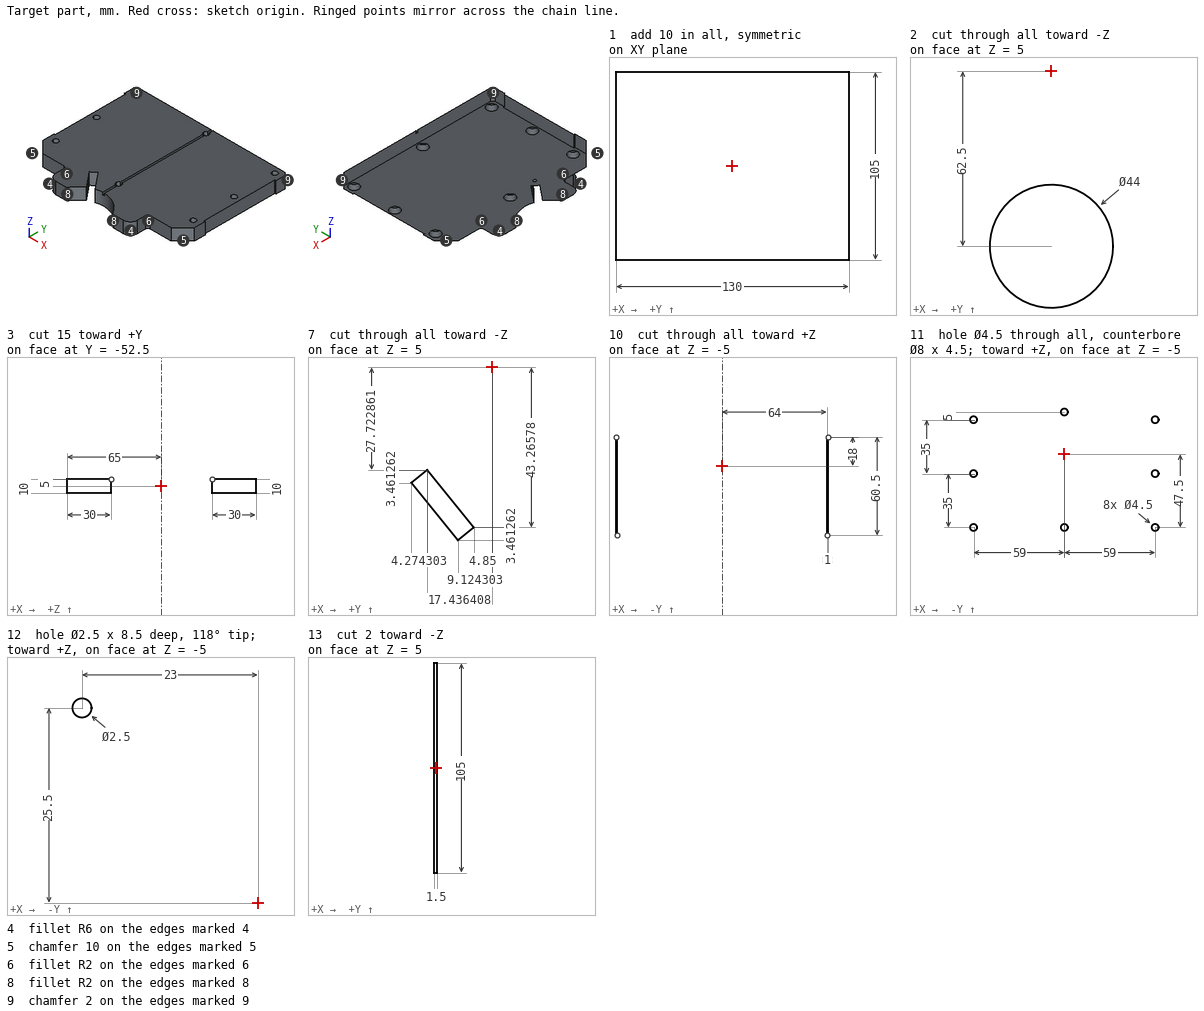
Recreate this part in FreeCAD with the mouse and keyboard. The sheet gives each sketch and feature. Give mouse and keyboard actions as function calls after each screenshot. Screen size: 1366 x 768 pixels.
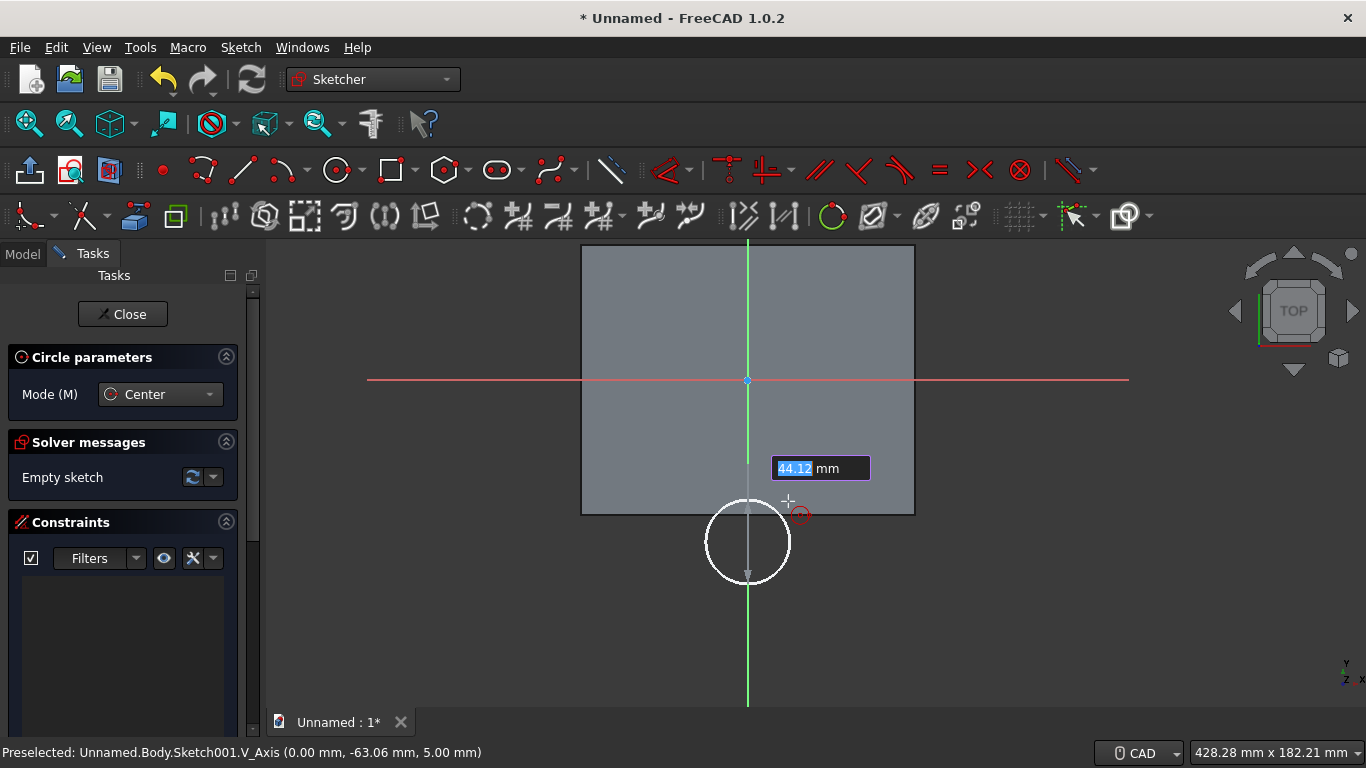
text(44)
key(Return)
key(Escape)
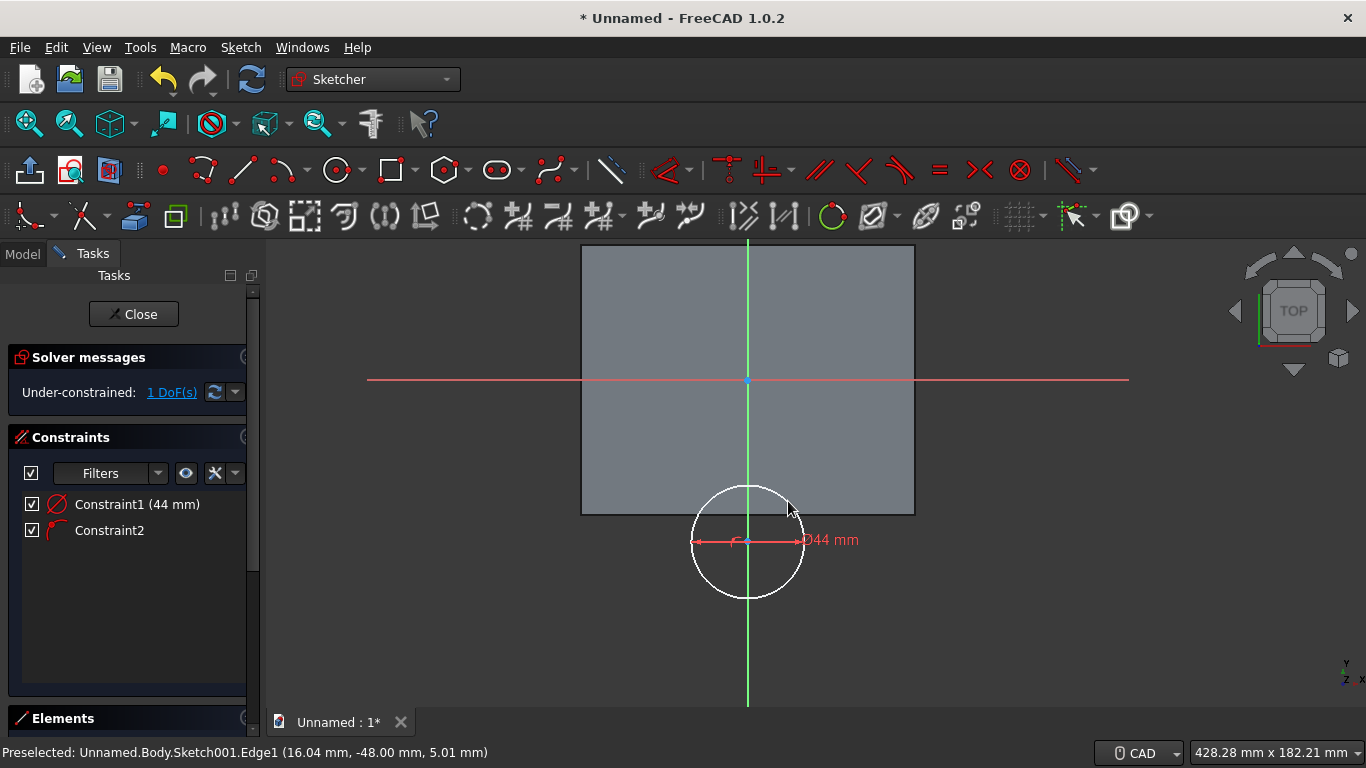
click(666, 170)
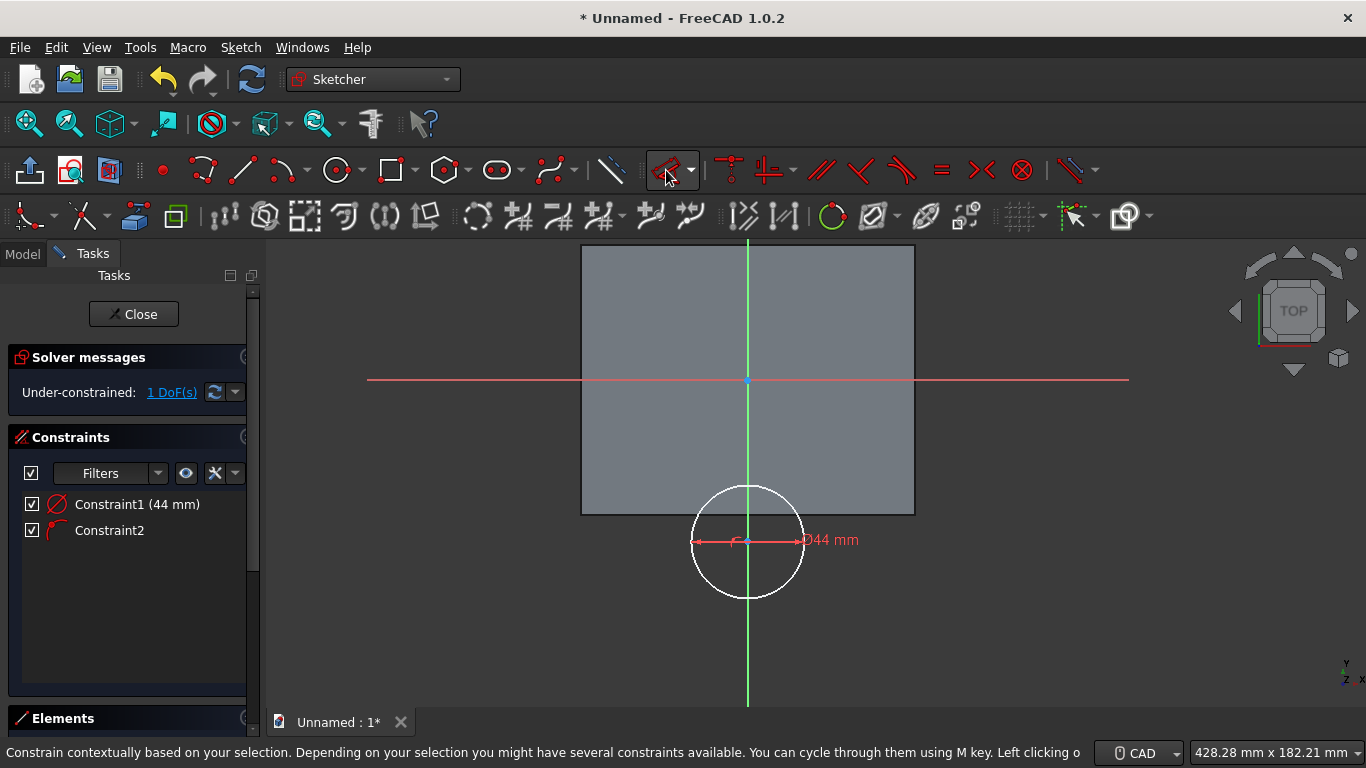
click(748, 542)
click(782, 461)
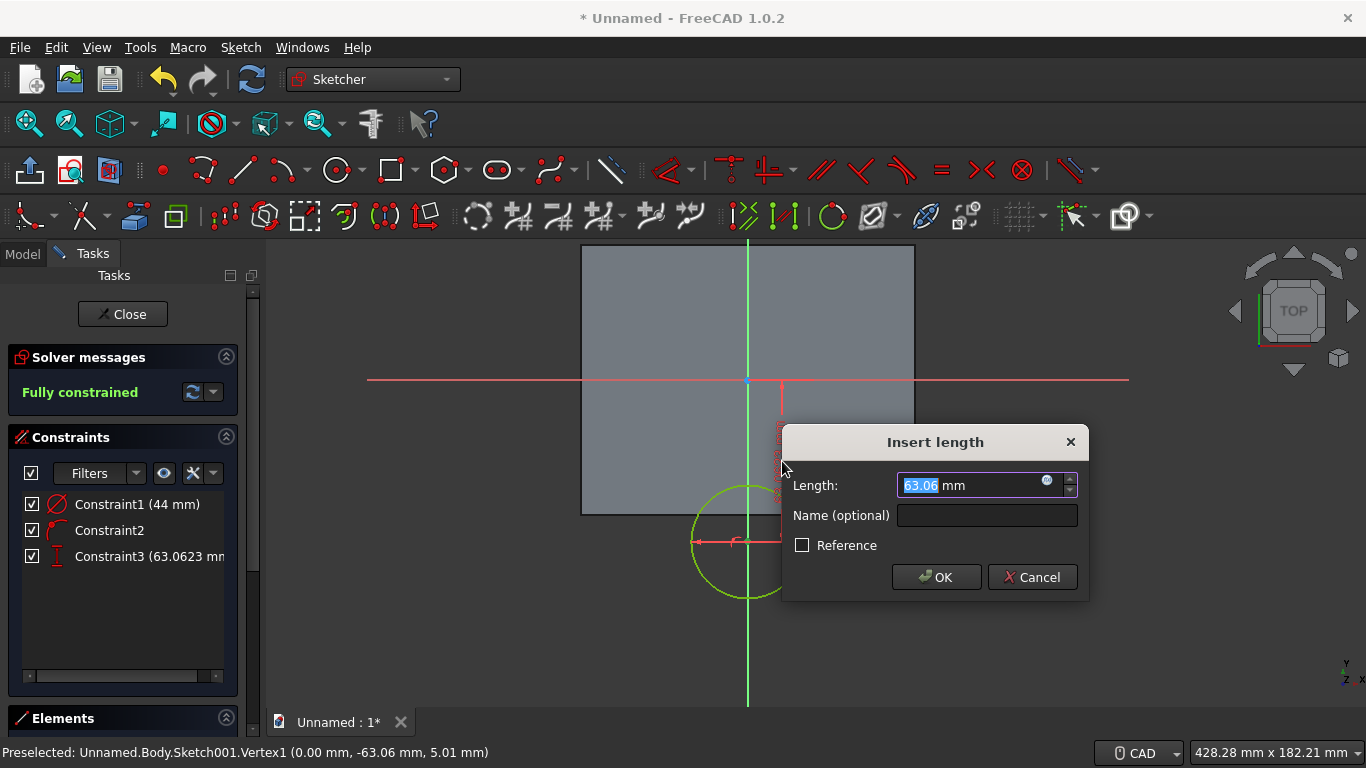
text(62.5)
key(Return)
key(Escape)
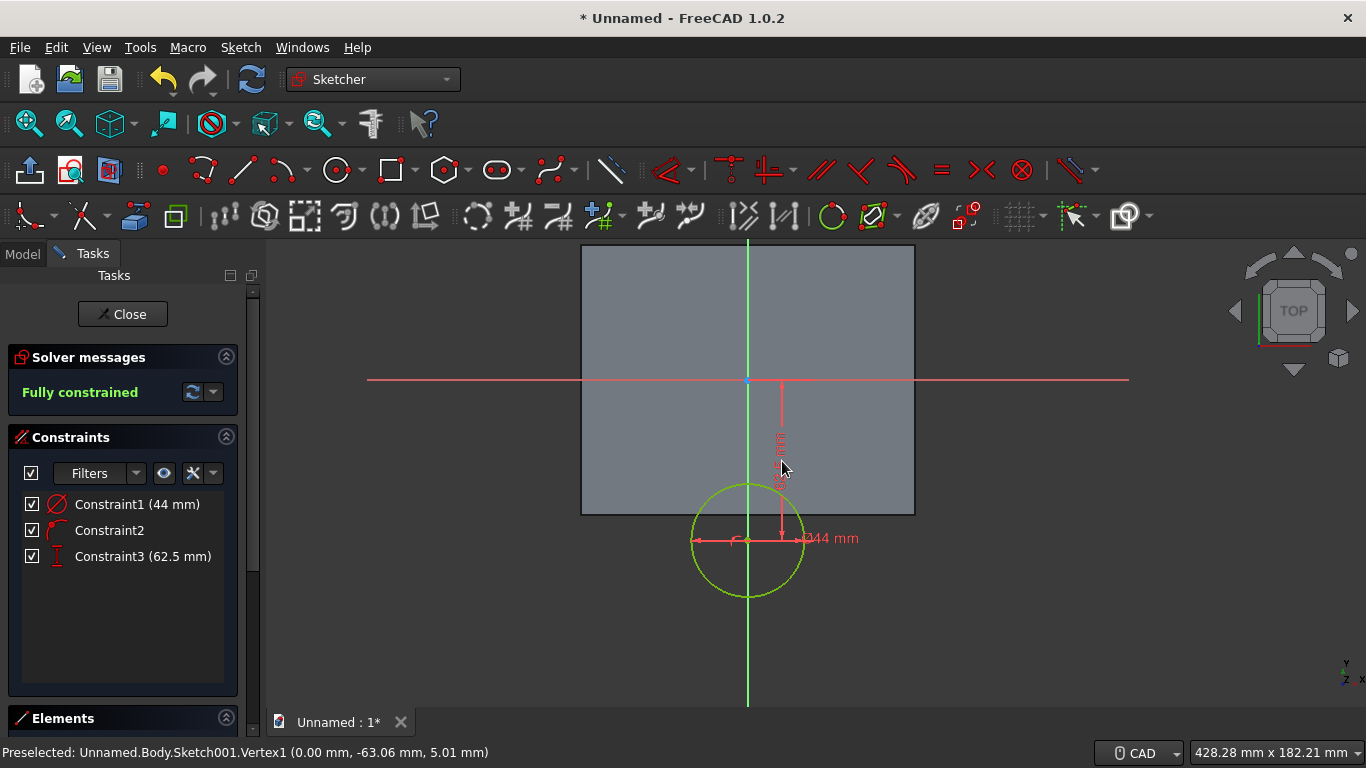
click(123, 314)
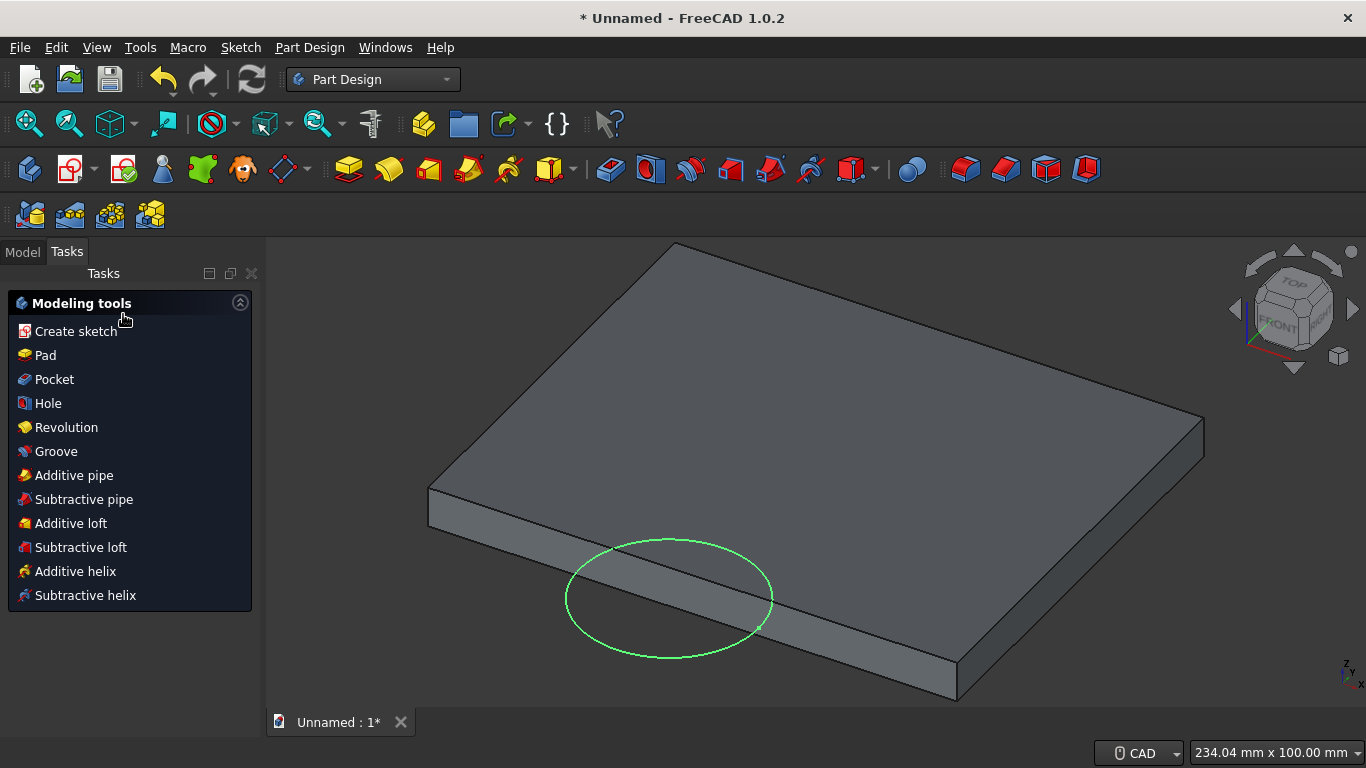
click(612, 170)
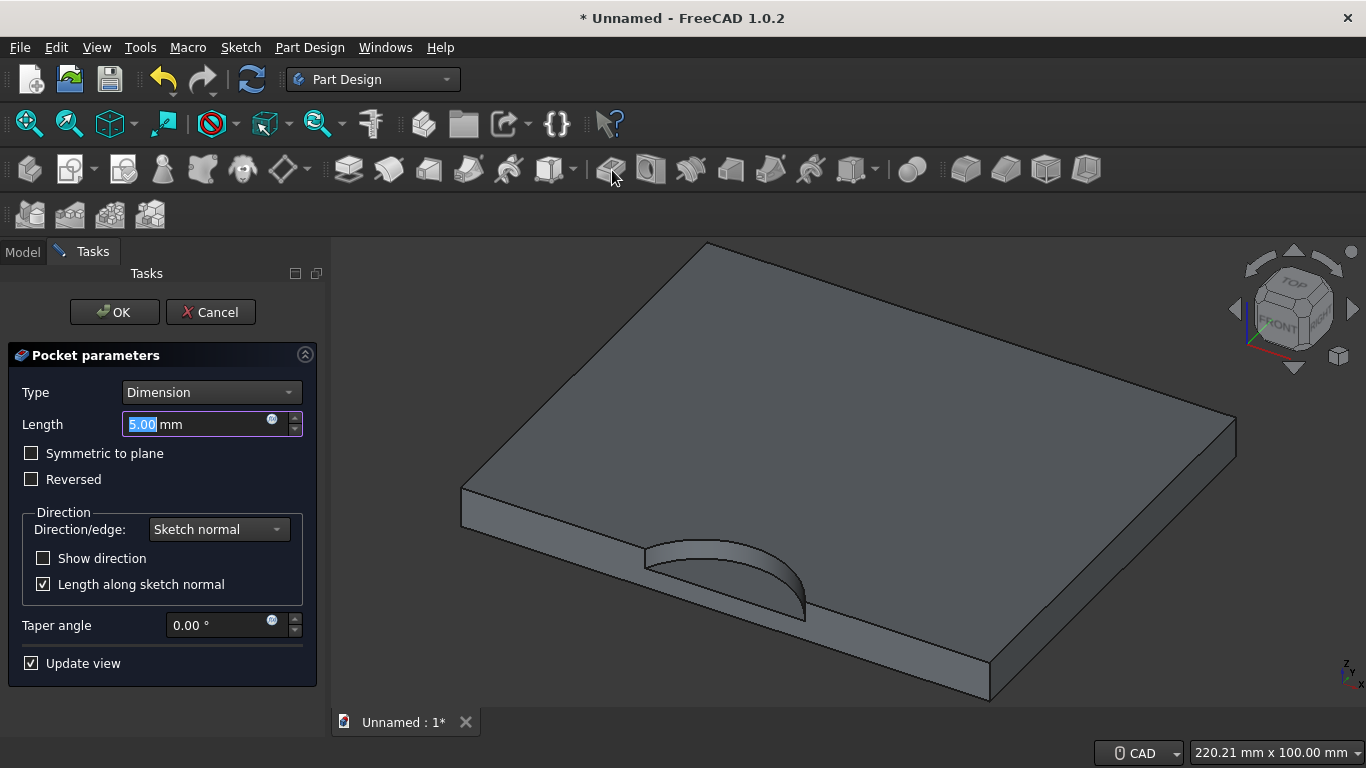
click(212, 392)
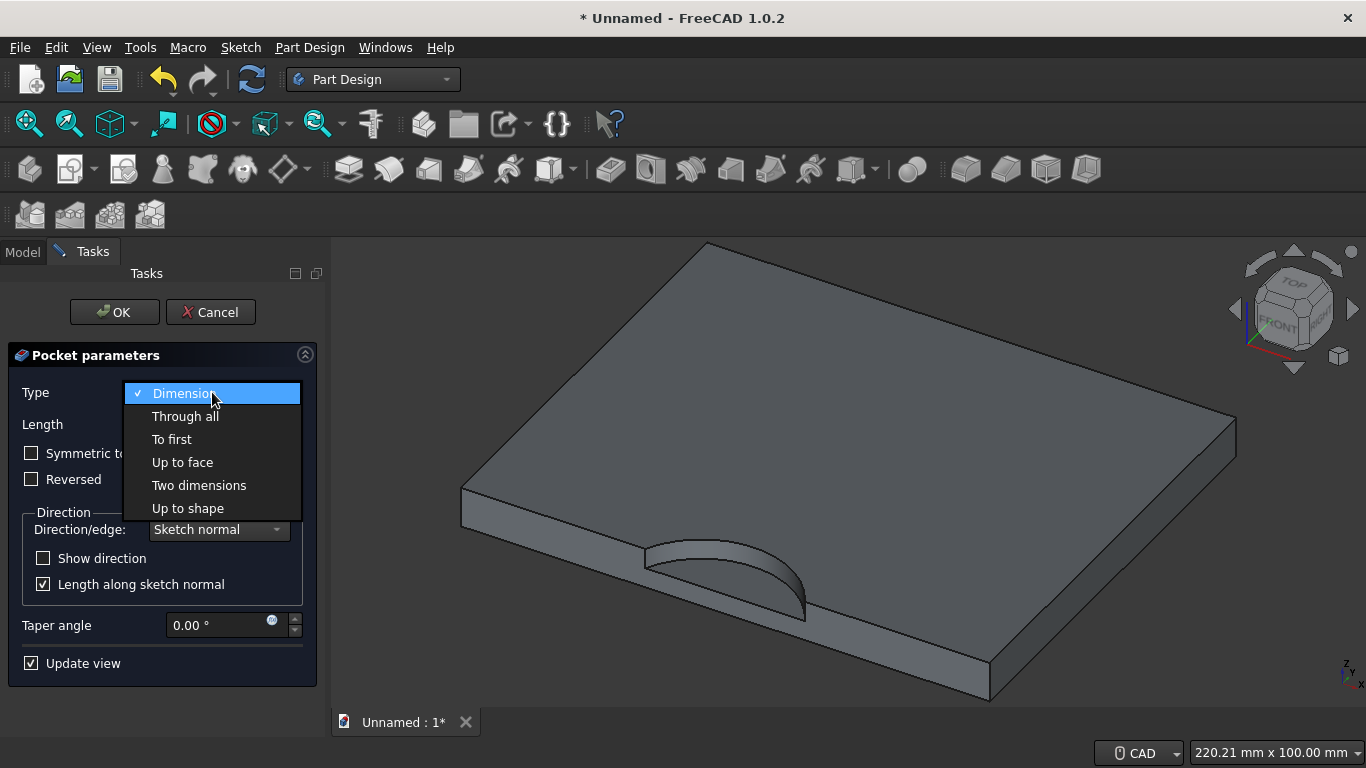
click(212, 416)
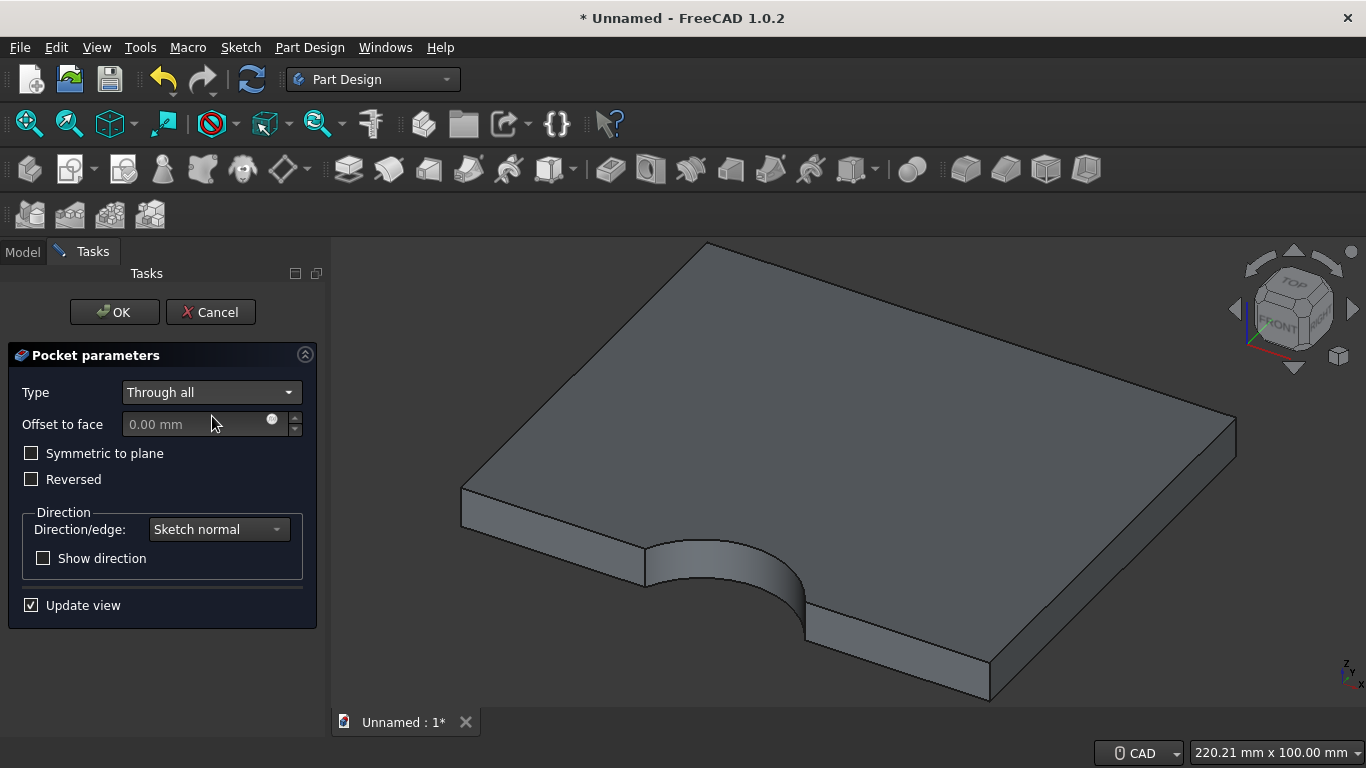
click(115, 312)